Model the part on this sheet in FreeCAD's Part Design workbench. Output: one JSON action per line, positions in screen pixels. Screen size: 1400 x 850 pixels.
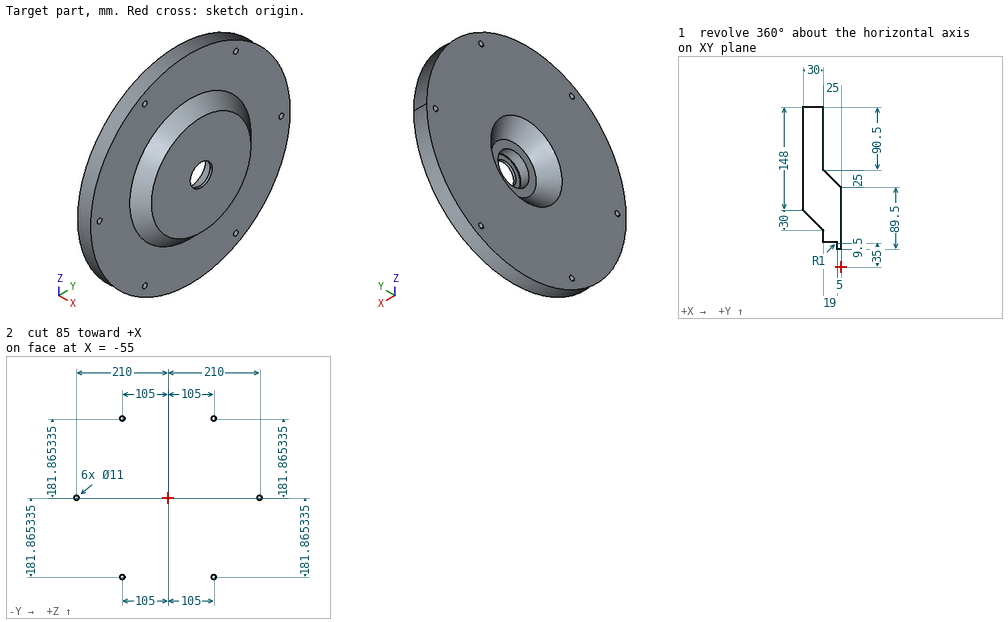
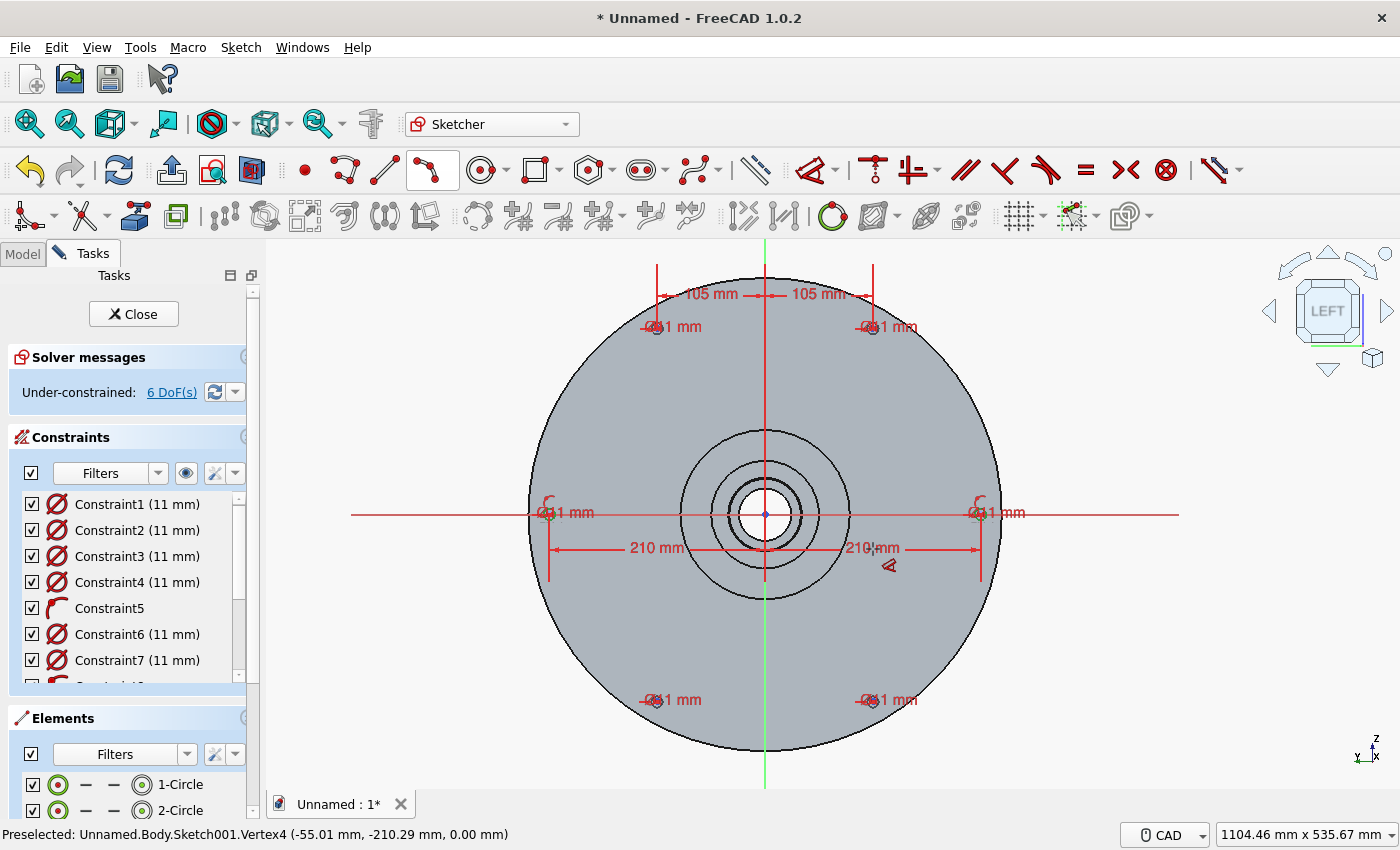
{"action": "left_click", "coordinate": [873, 702]}
{"action": "left_click", "coordinate": [819, 736]}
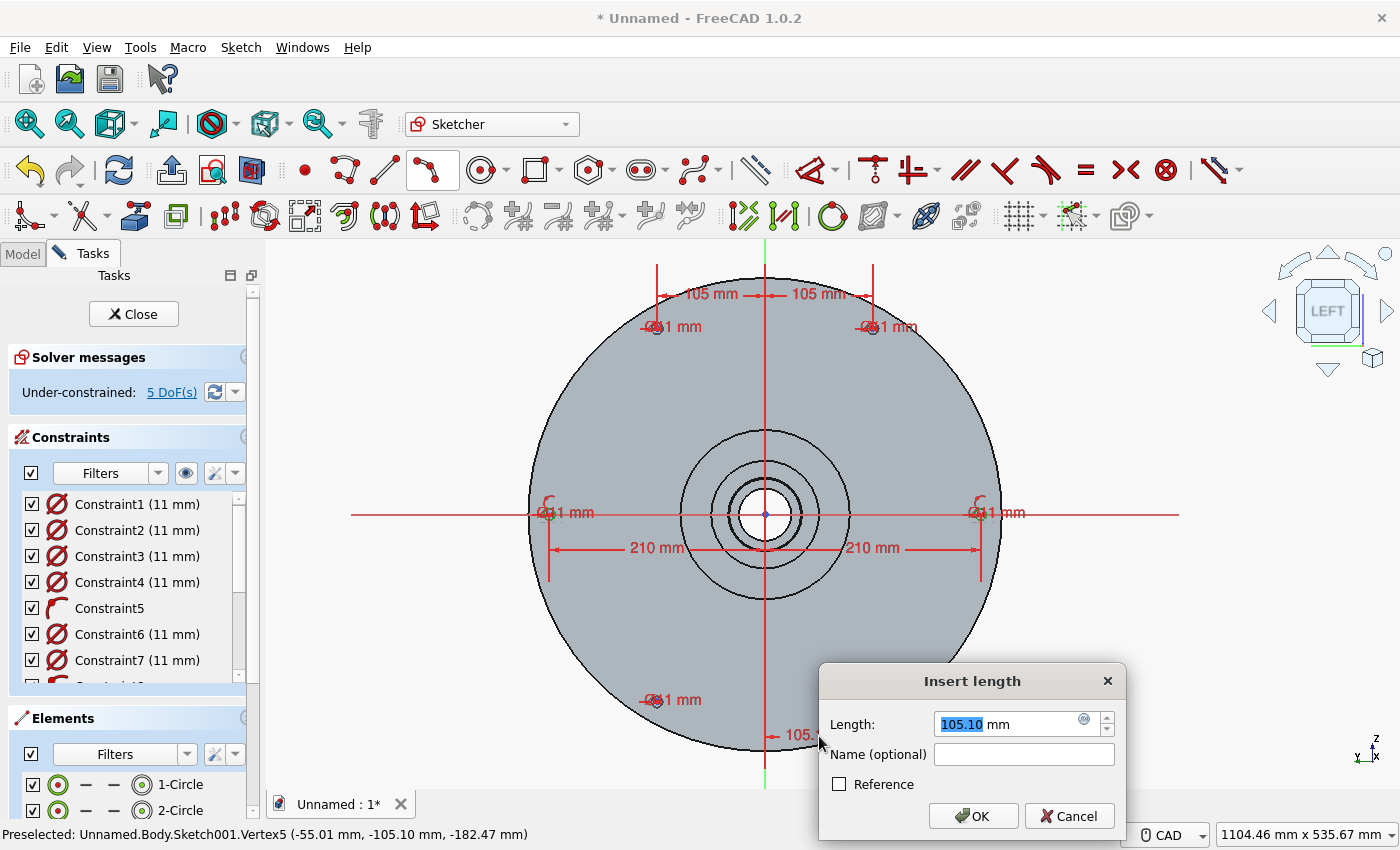
{"action": "type", "text": "105"}
{"action": "key", "text": "Return"}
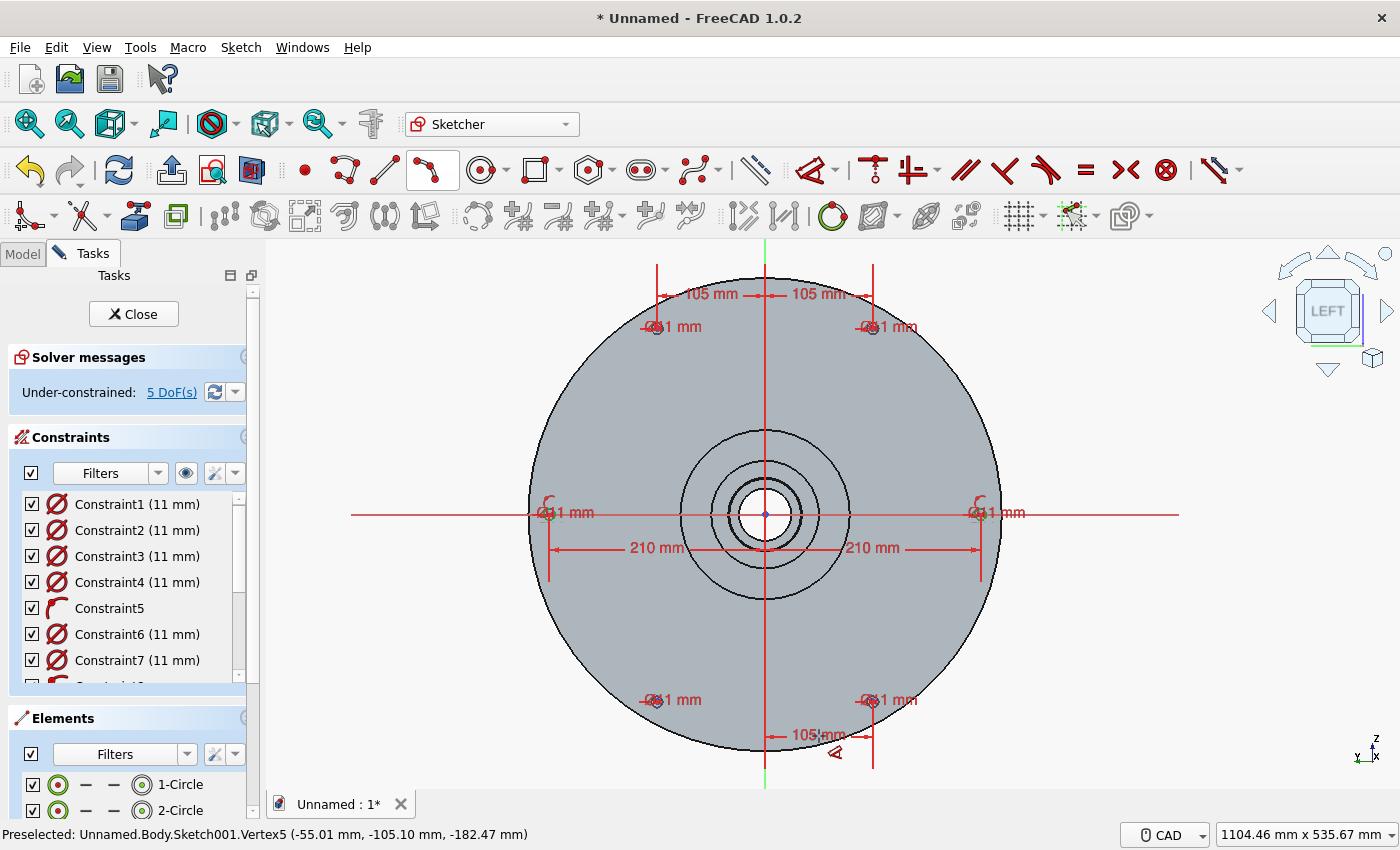
{"action": "left_click", "coordinate": [657, 702]}
{"action": "left_click", "coordinate": [711, 736]}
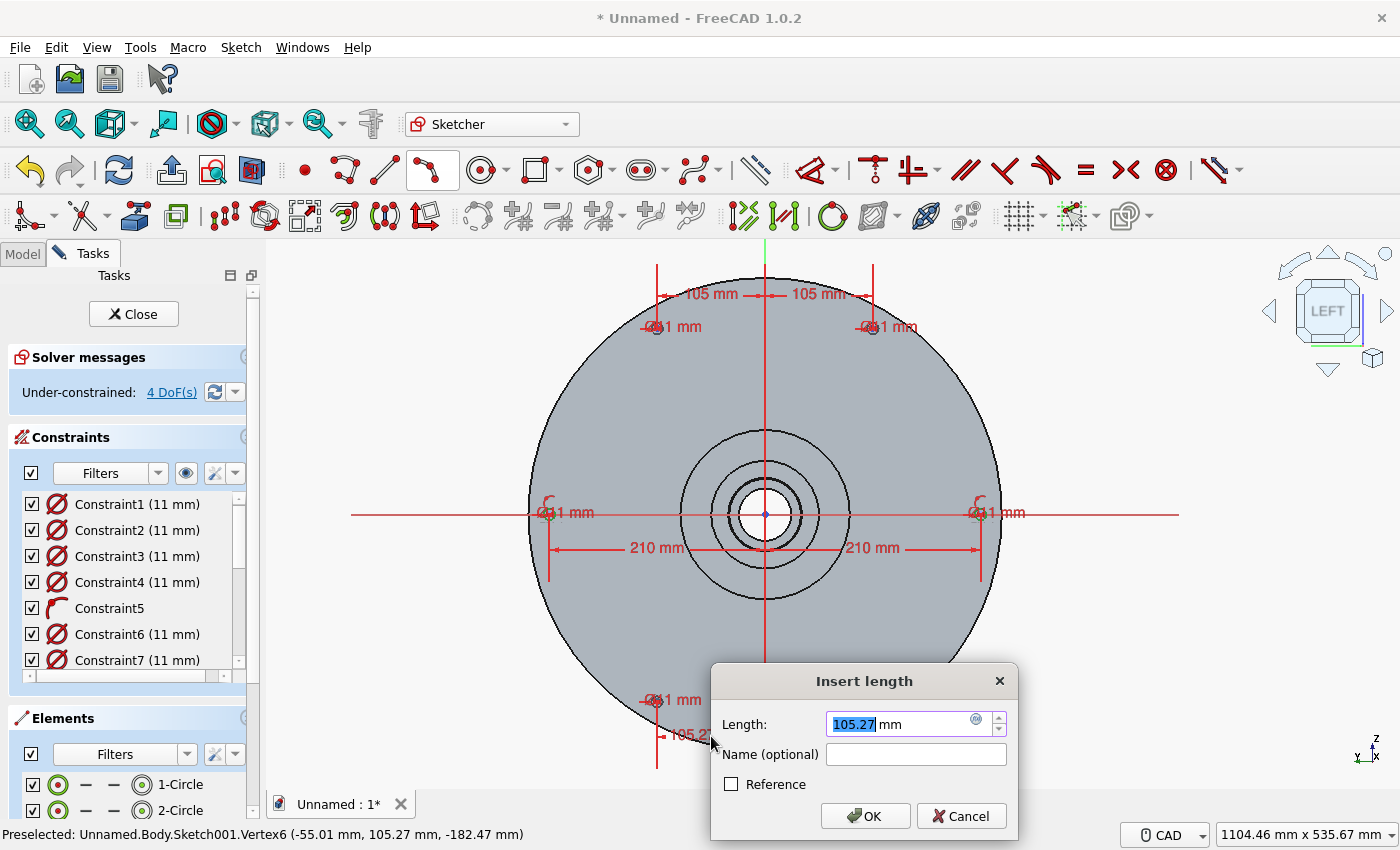
{"action": "type", "text": "105"}
{"action": "key", "text": "Return"}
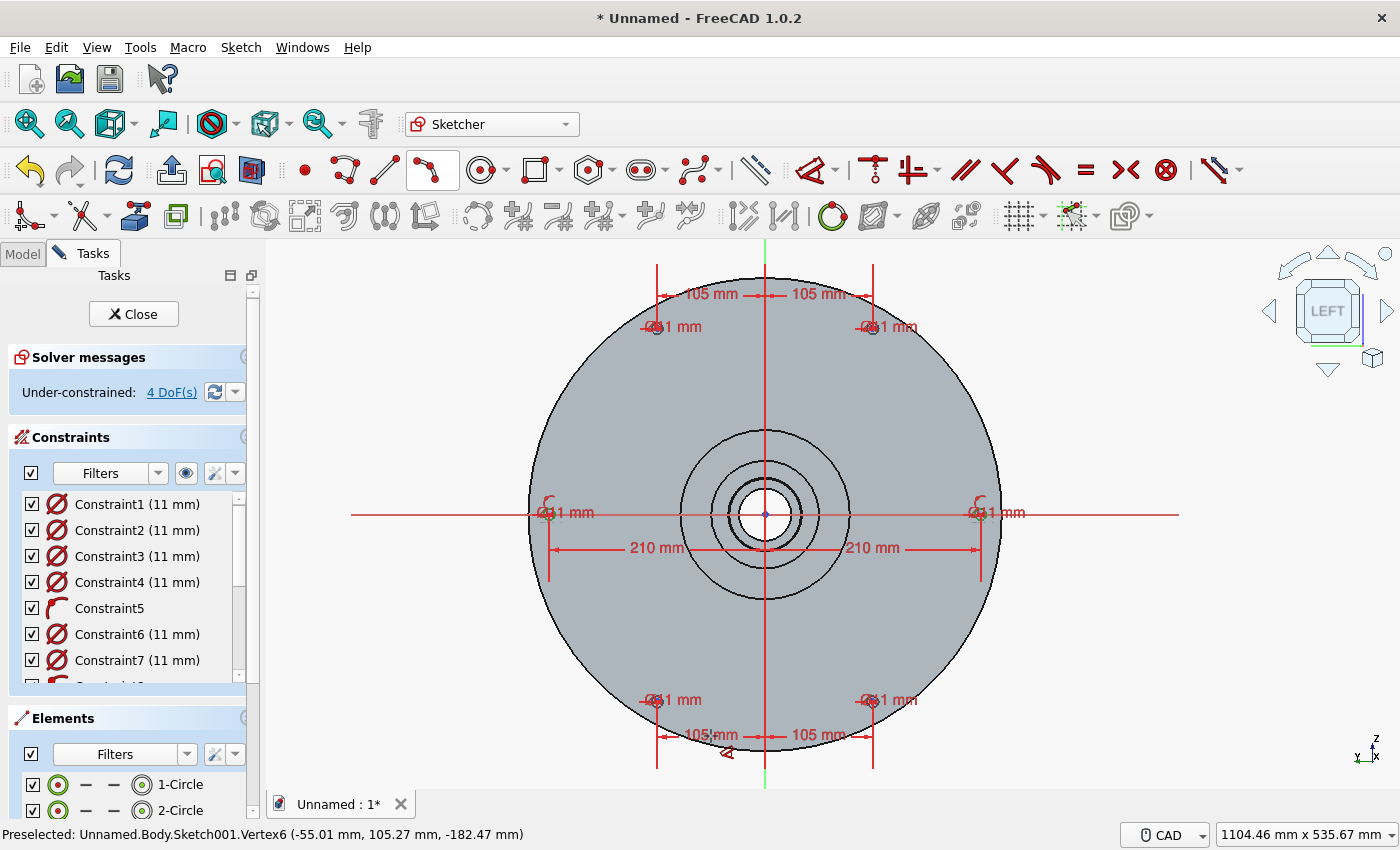
{"action": "left_click", "coordinate": [657, 329]}
{"action": "left_click", "coordinate": [623, 422]}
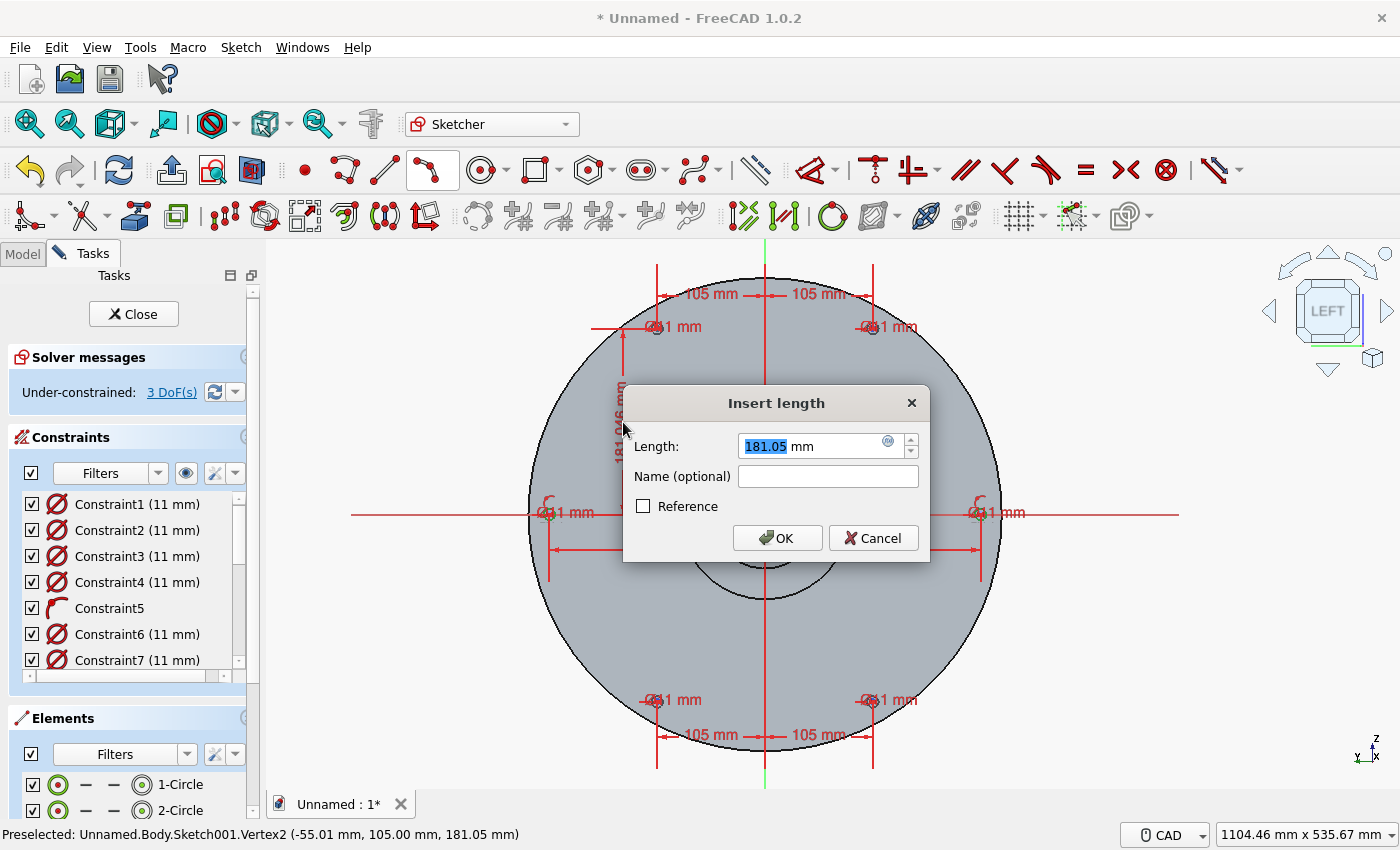
{"action": "type", "text": "181.865335"}
{"action": "key", "text": "Return"}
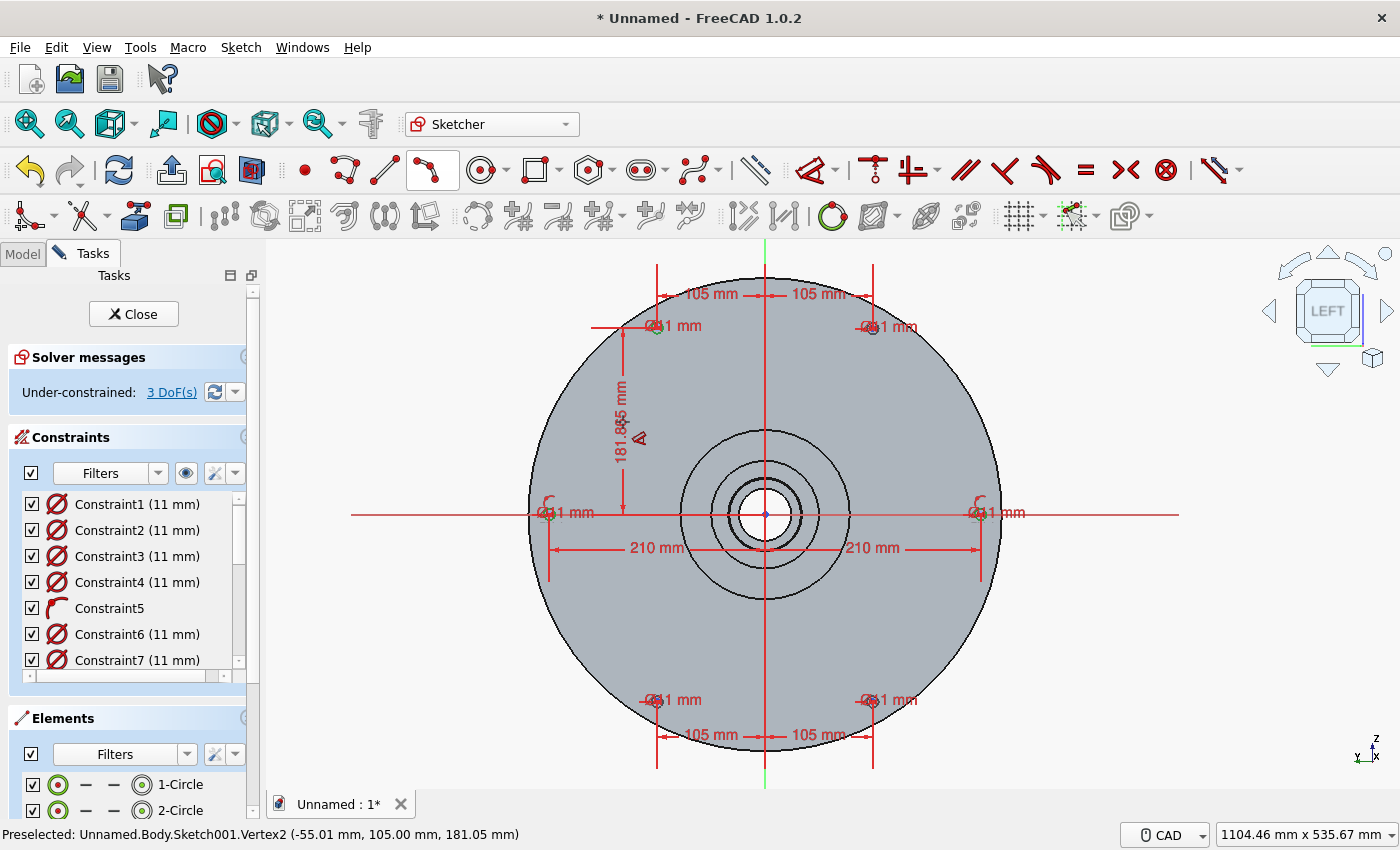
{"action": "left_click", "coordinate": [873, 329]}
{"action": "left_click", "coordinate": [907, 422]}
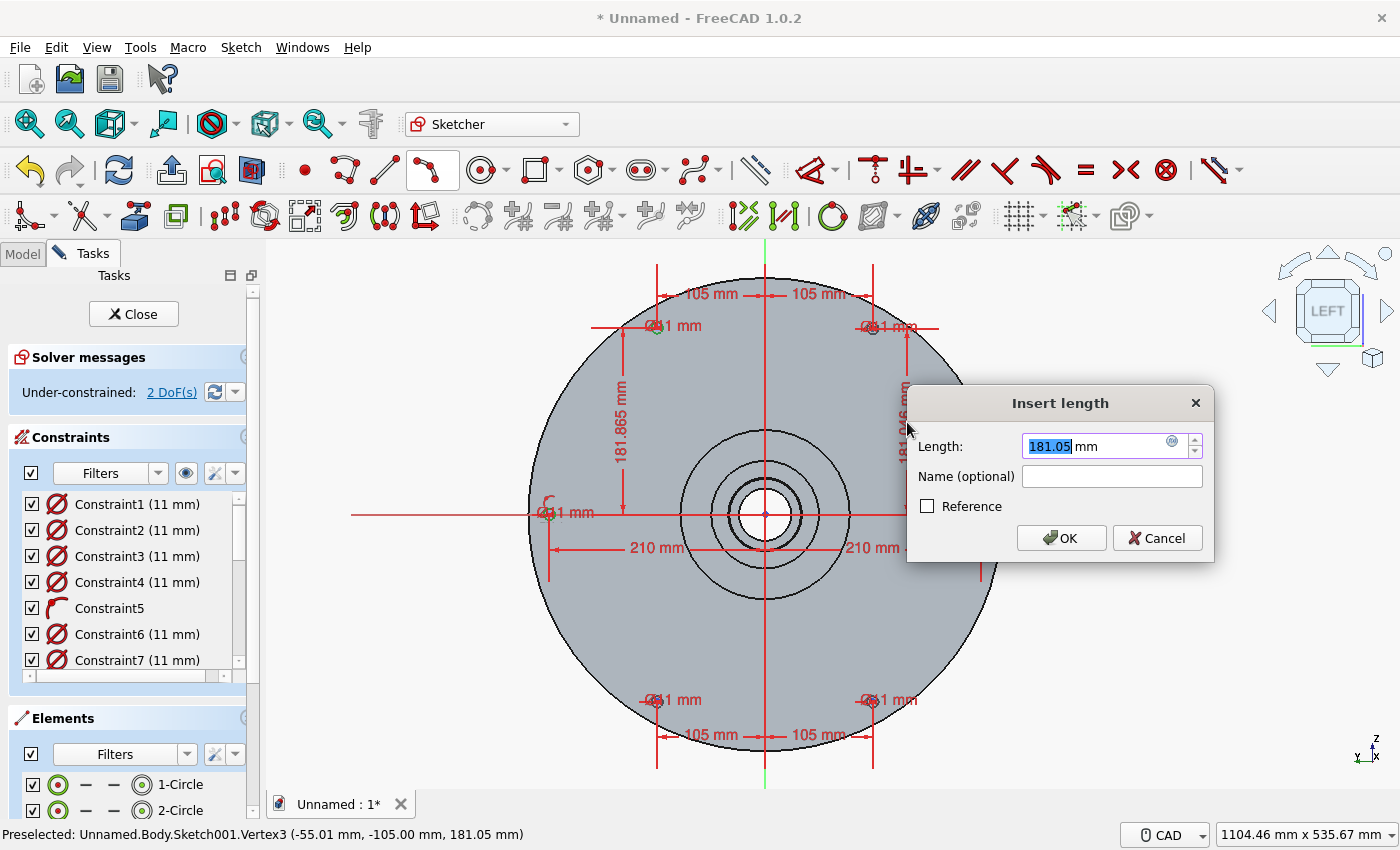
{"action": "type", "text": "181.865335"}
{"action": "key", "text": "Return"}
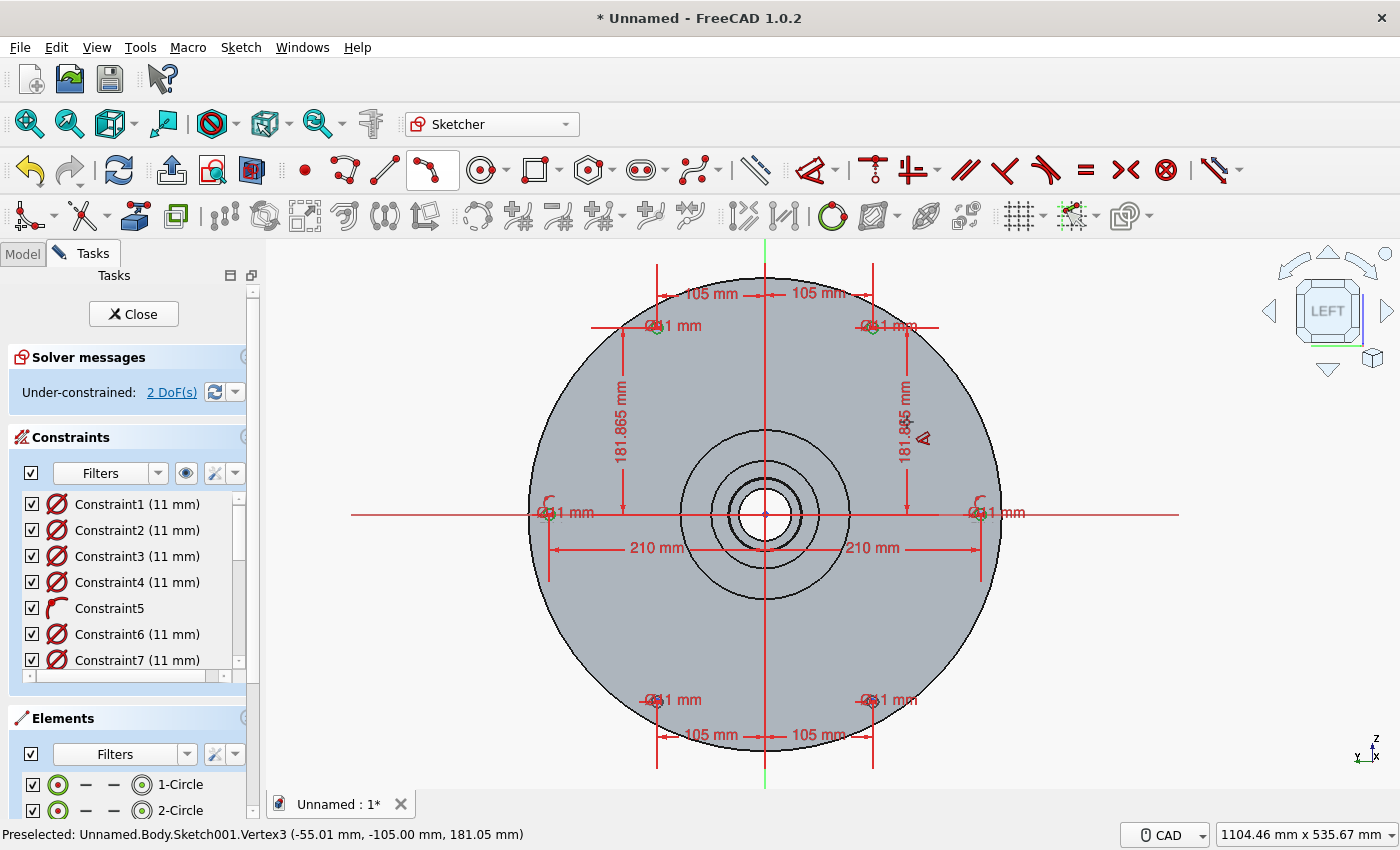
{"action": "left_click", "coordinate": [873, 702]}
{"action": "left_click", "coordinate": [907, 608]}